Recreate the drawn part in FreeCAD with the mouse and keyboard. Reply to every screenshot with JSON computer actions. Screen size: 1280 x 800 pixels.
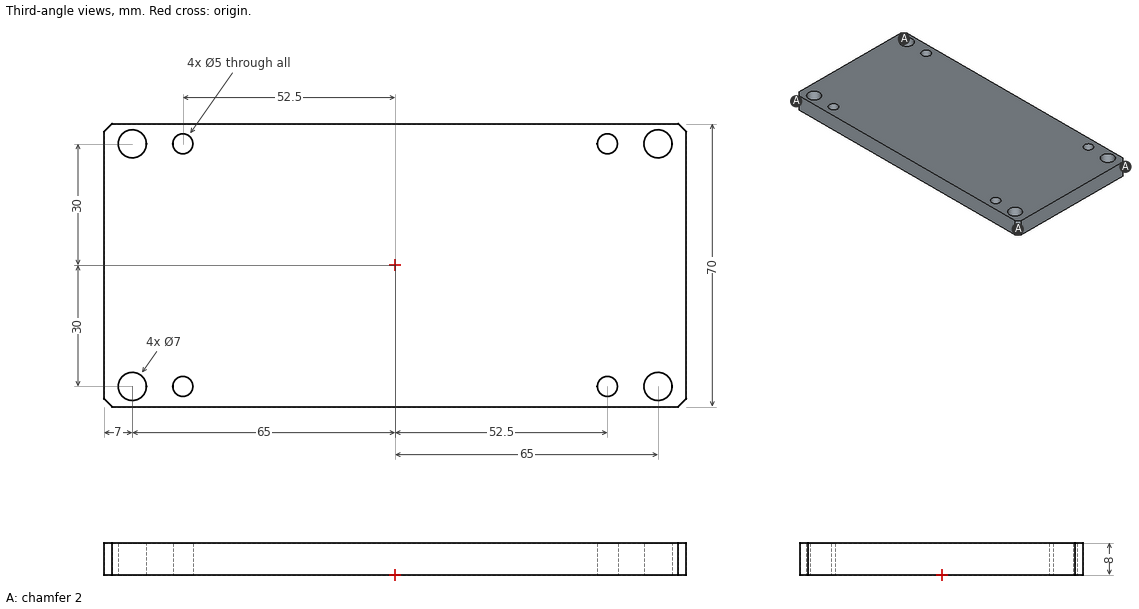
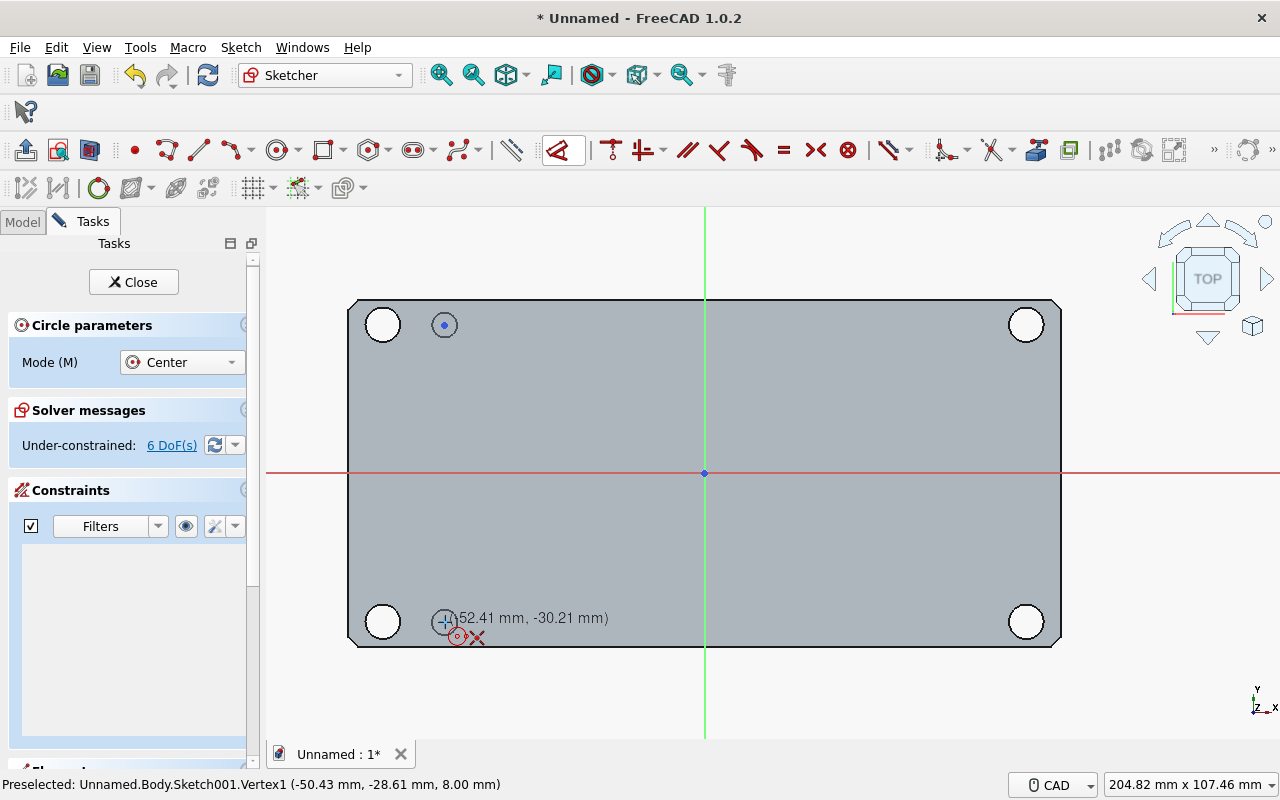
{"action": "scroll", "coordinate": [964, 622], "scroll_direction": "up", "scroll_amount": 4}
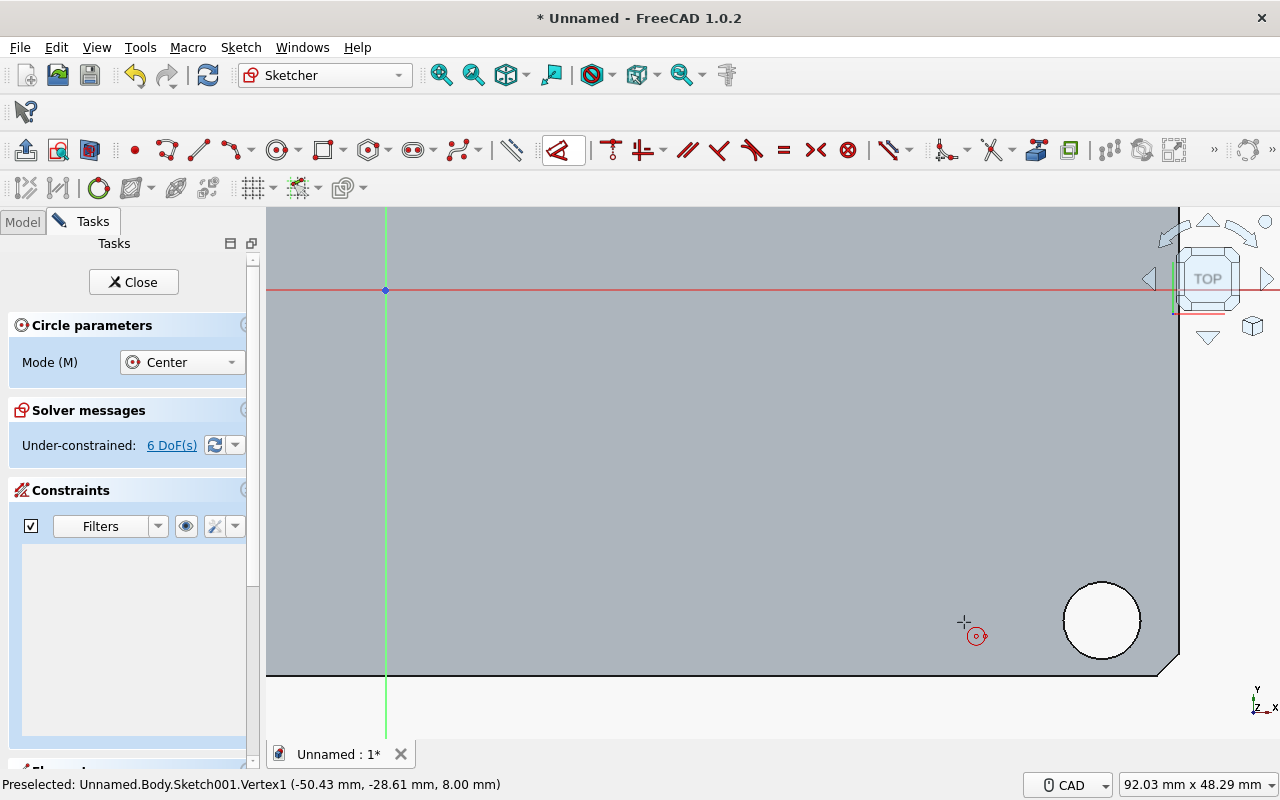
{"action": "left_click", "coordinate": [964, 621]}
{"action": "left_click", "coordinate": [984, 601]}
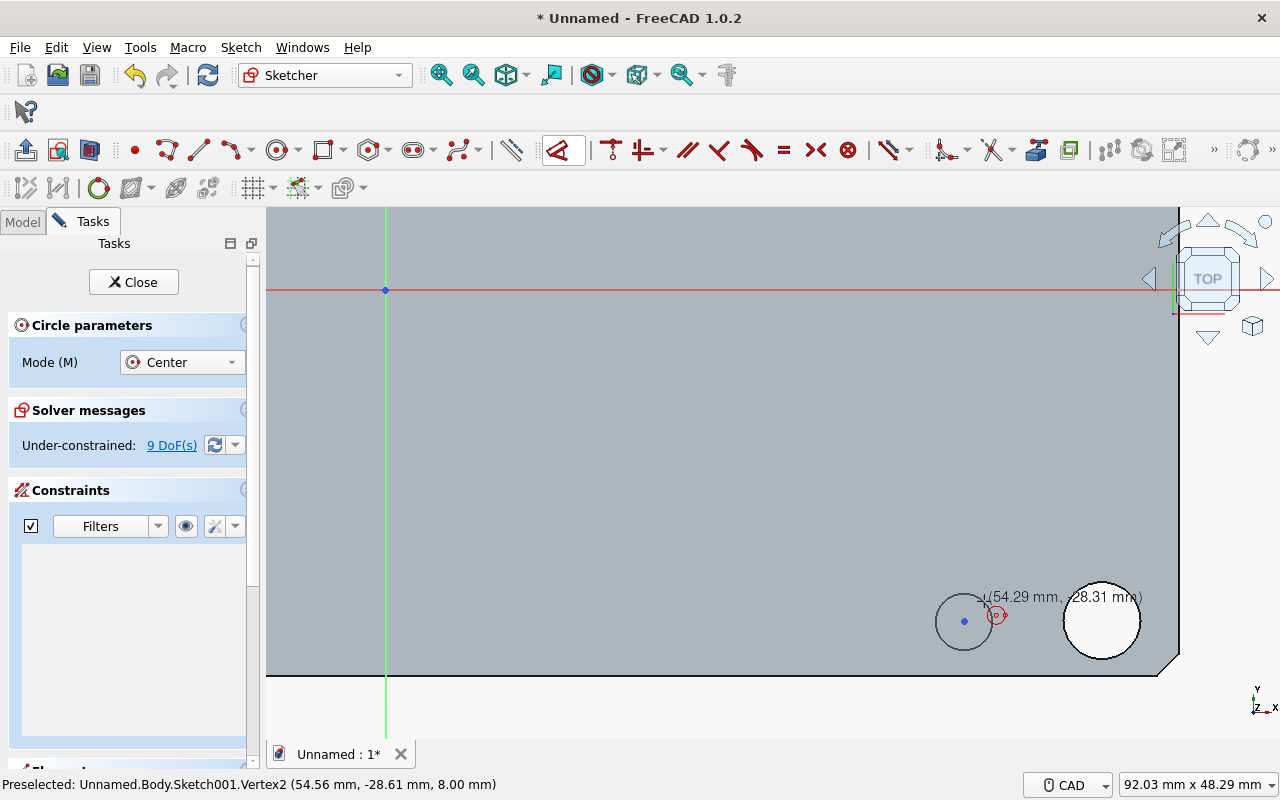
{"action": "scroll", "coordinate": [965, 622], "scroll_direction": "down", "scroll_amount": 4}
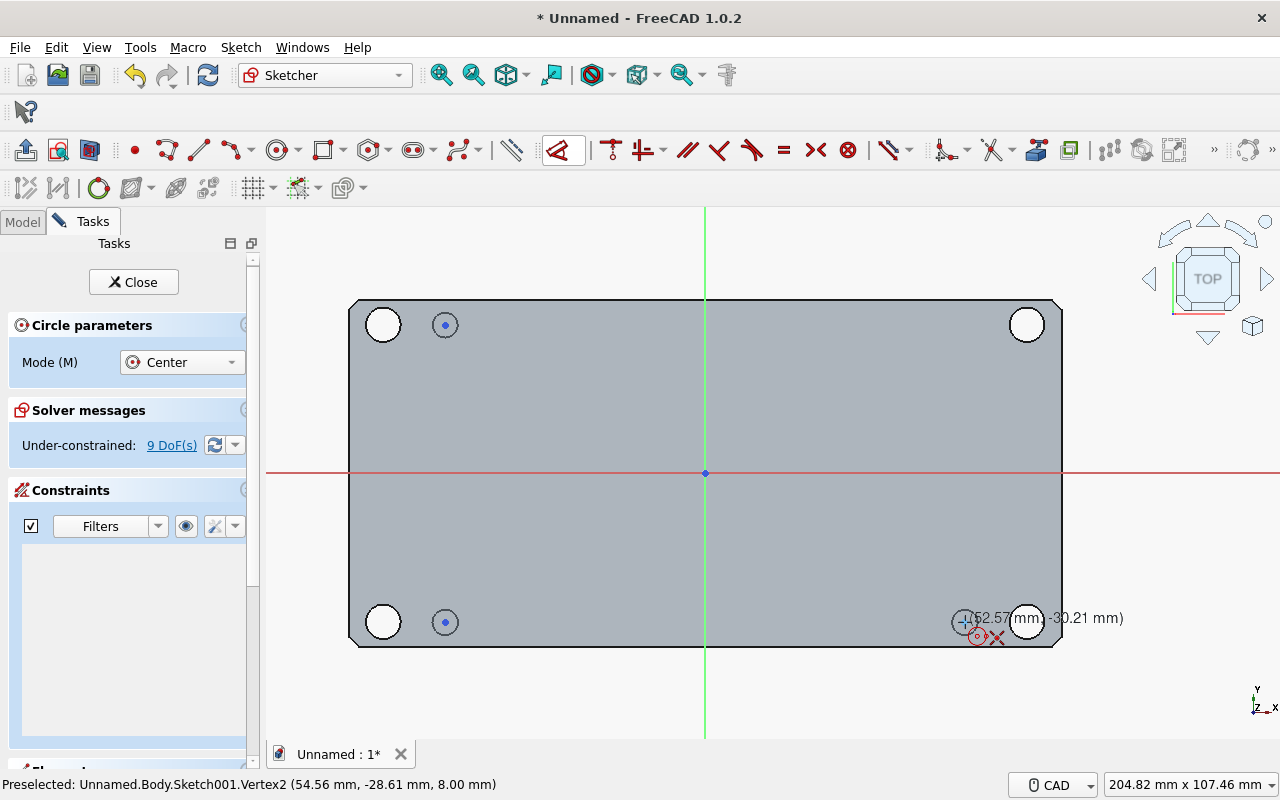
{"action": "scroll", "coordinate": [965, 325], "scroll_direction": "up", "scroll_amount": 4}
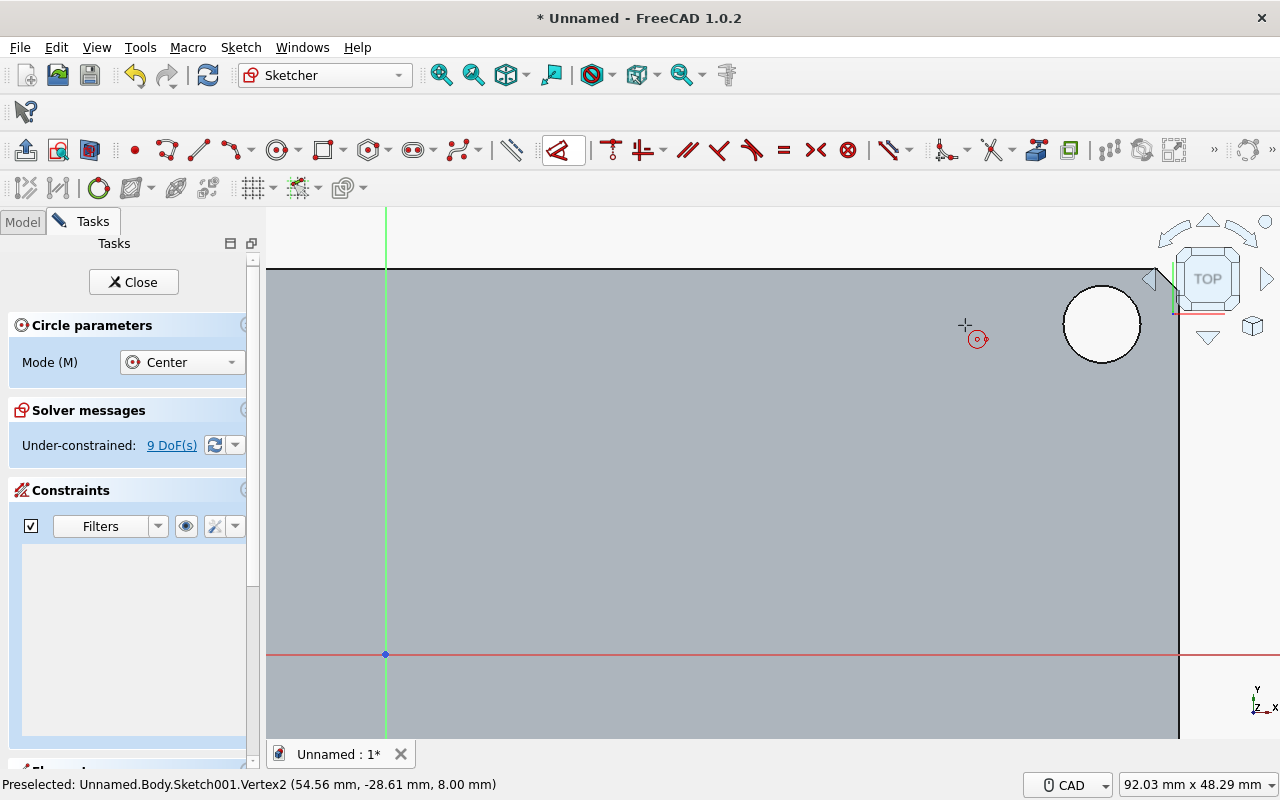
{"action": "left_click", "coordinate": [964, 324]}
{"action": "left_click", "coordinate": [984, 305]}
{"action": "key", "text": "Escape"}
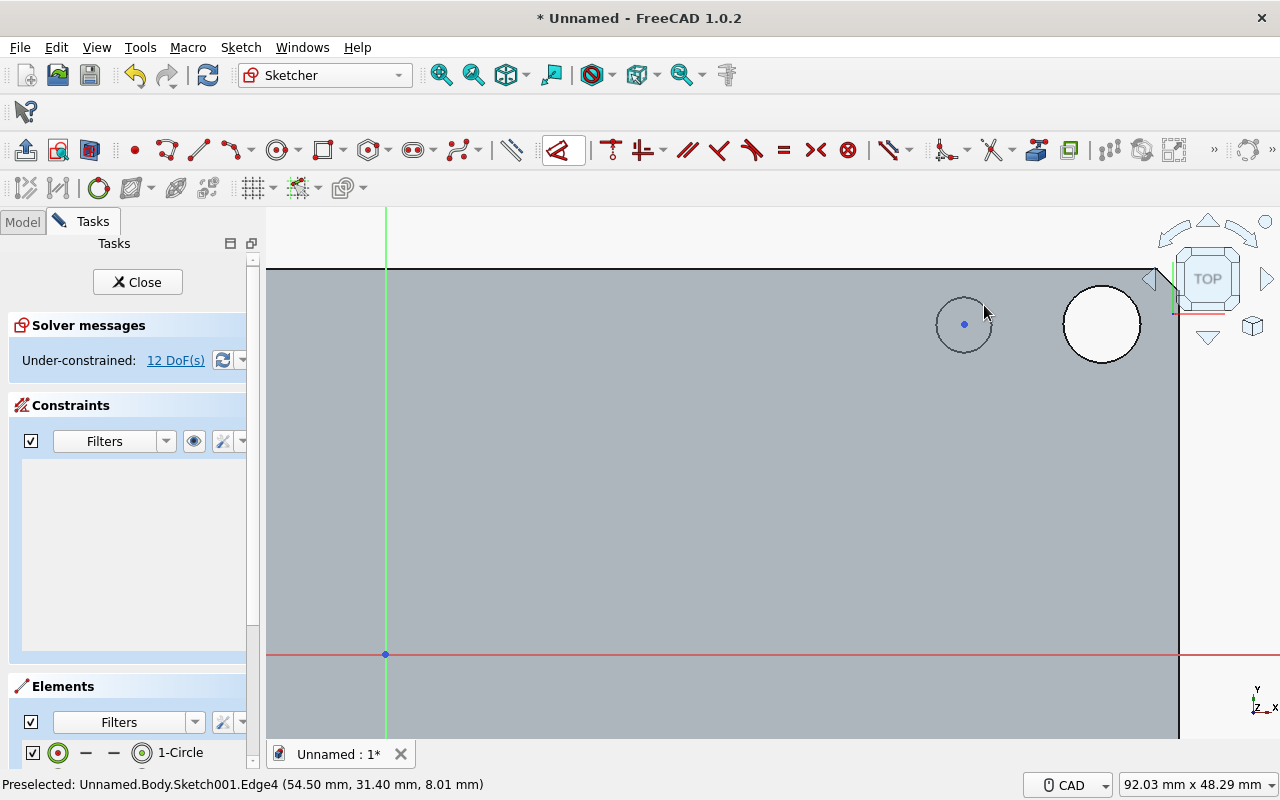
{"action": "scroll", "coordinate": [965, 325], "scroll_direction": "down", "scroll_amount": 4}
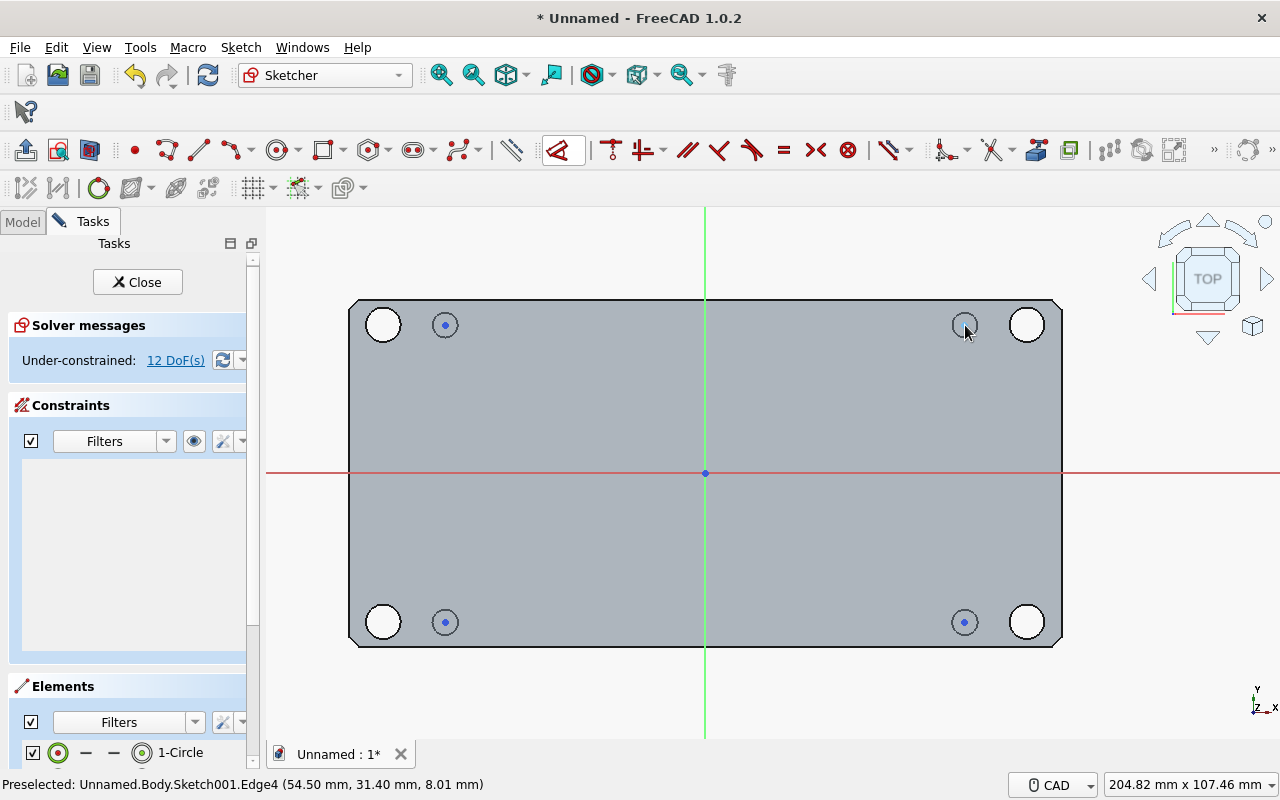
{"action": "left_click", "coordinate": [454, 316]}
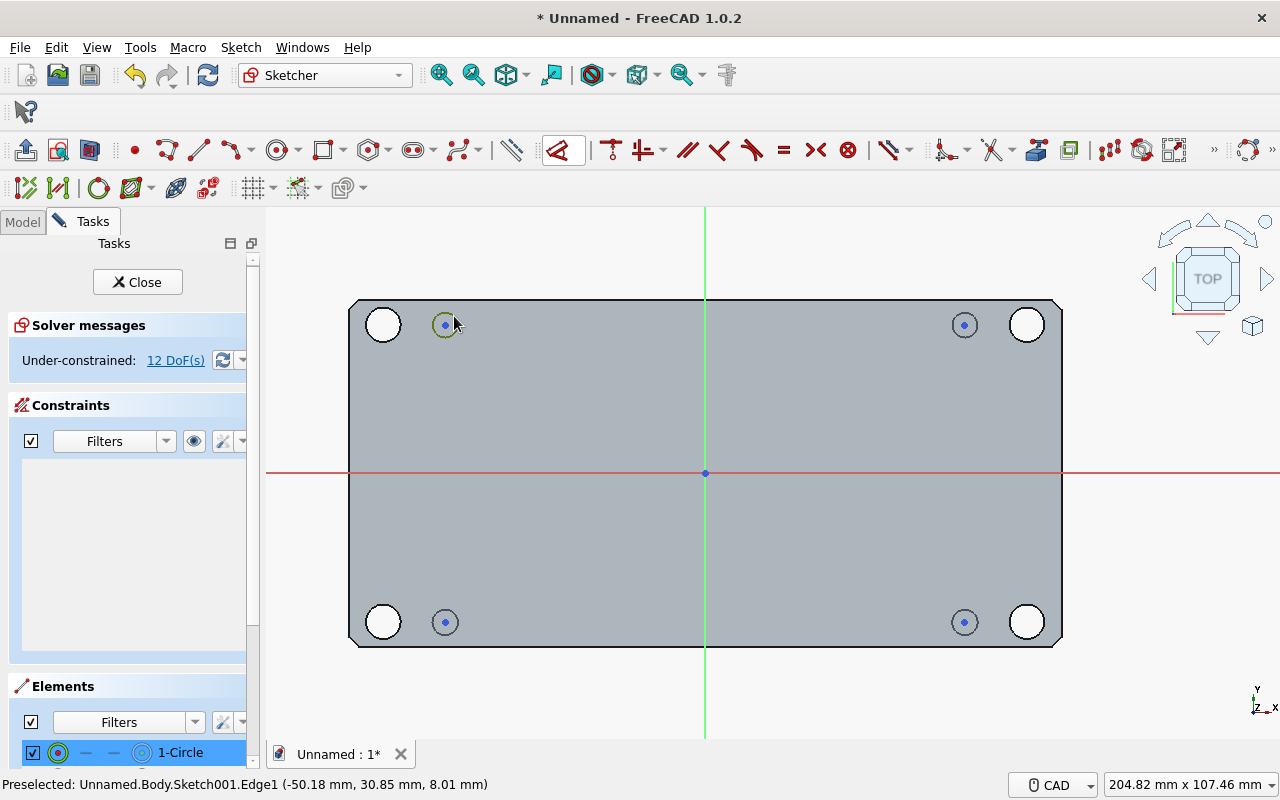
{"action": "left_click", "coordinate": [454, 613]}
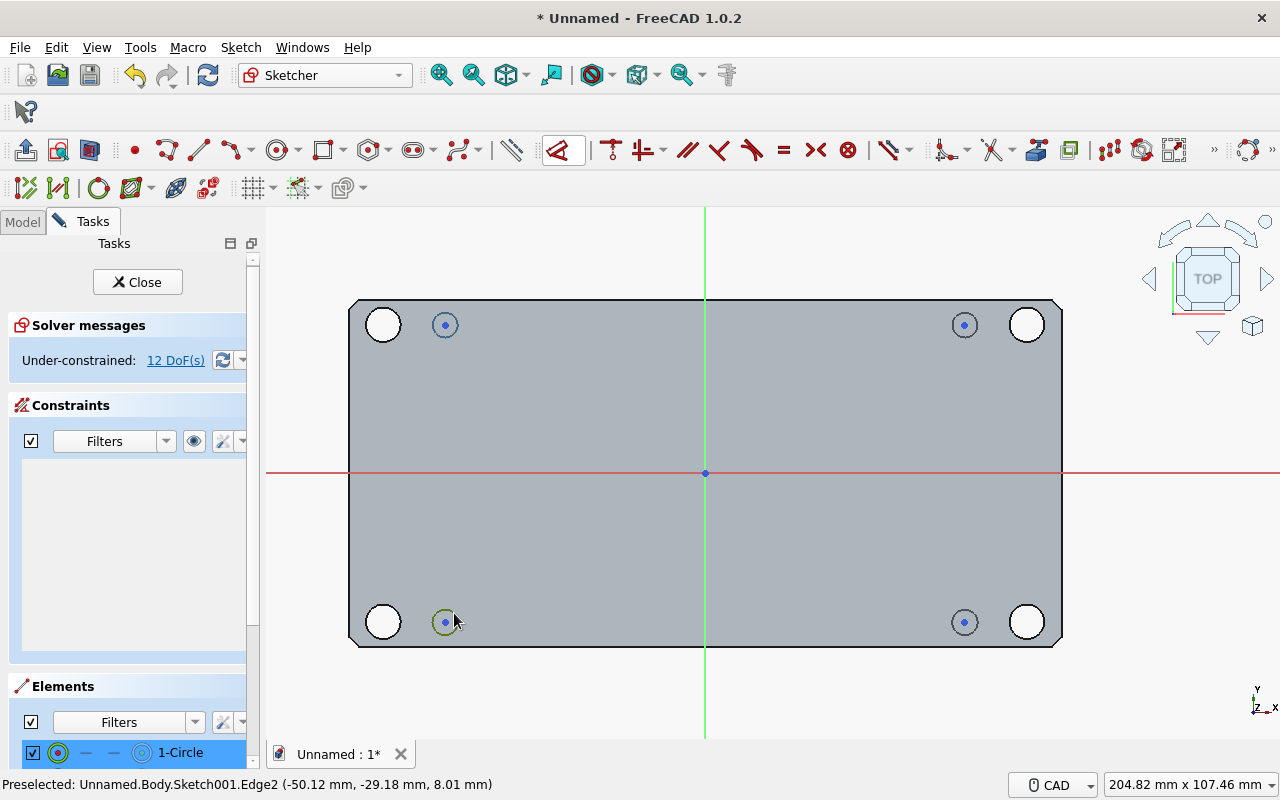
{"action": "left_click", "coordinate": [974, 613]}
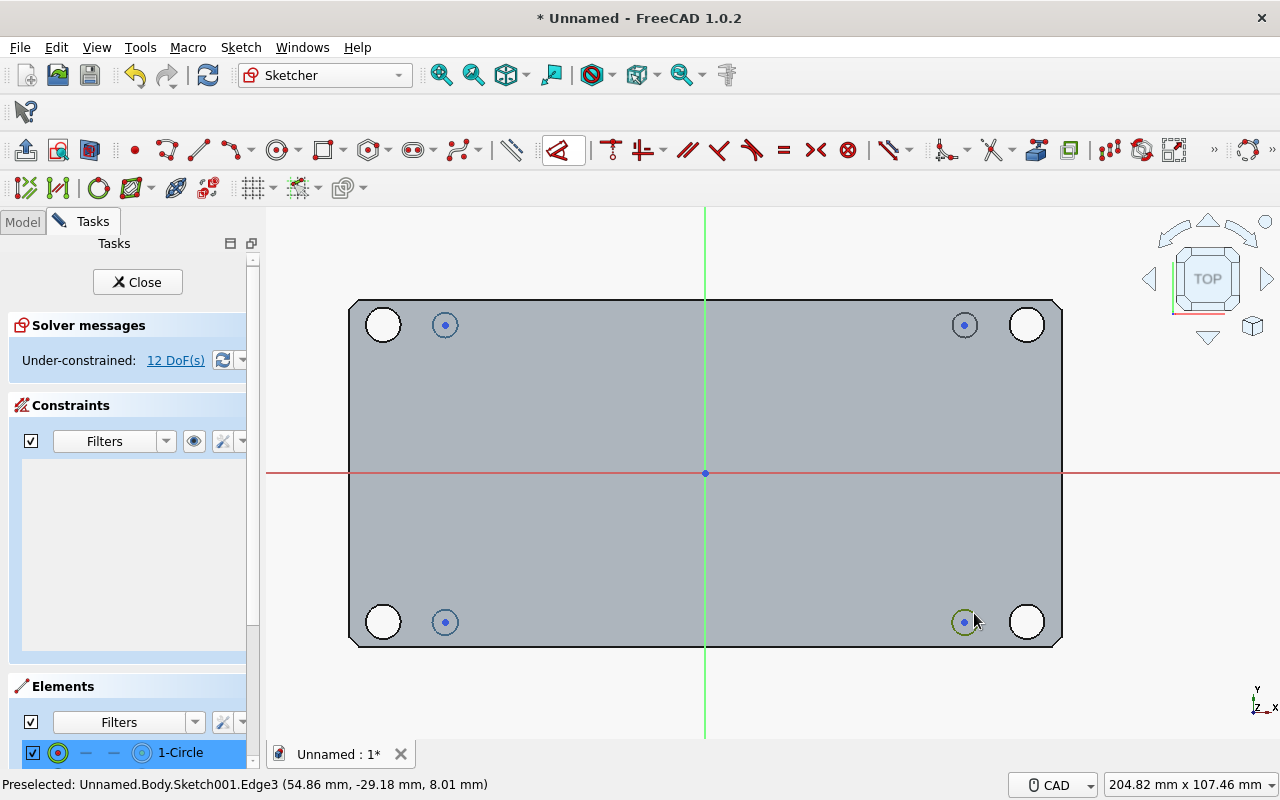
{"action": "left_click", "coordinate": [974, 316]}